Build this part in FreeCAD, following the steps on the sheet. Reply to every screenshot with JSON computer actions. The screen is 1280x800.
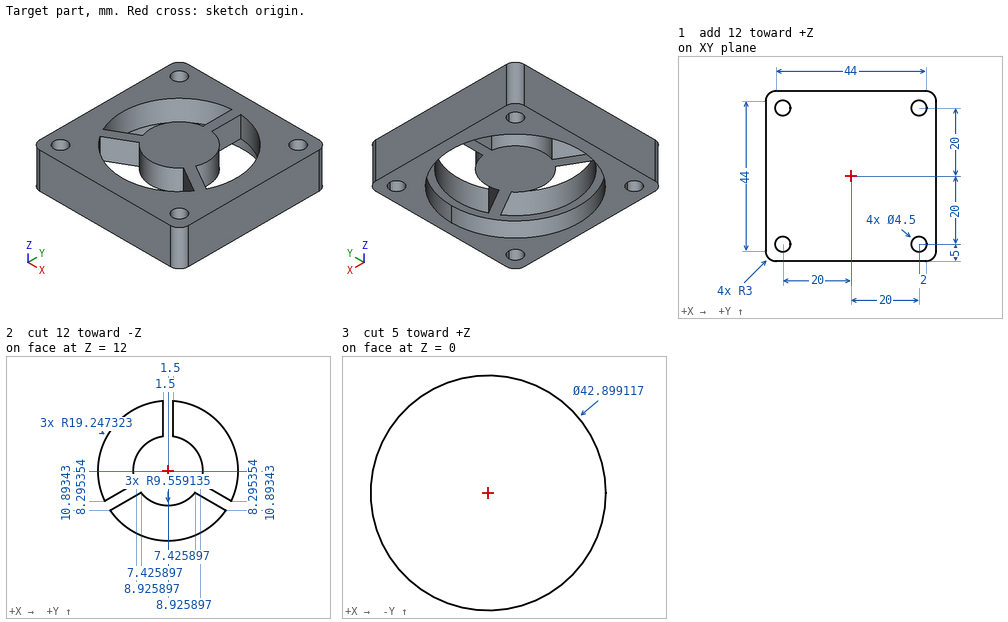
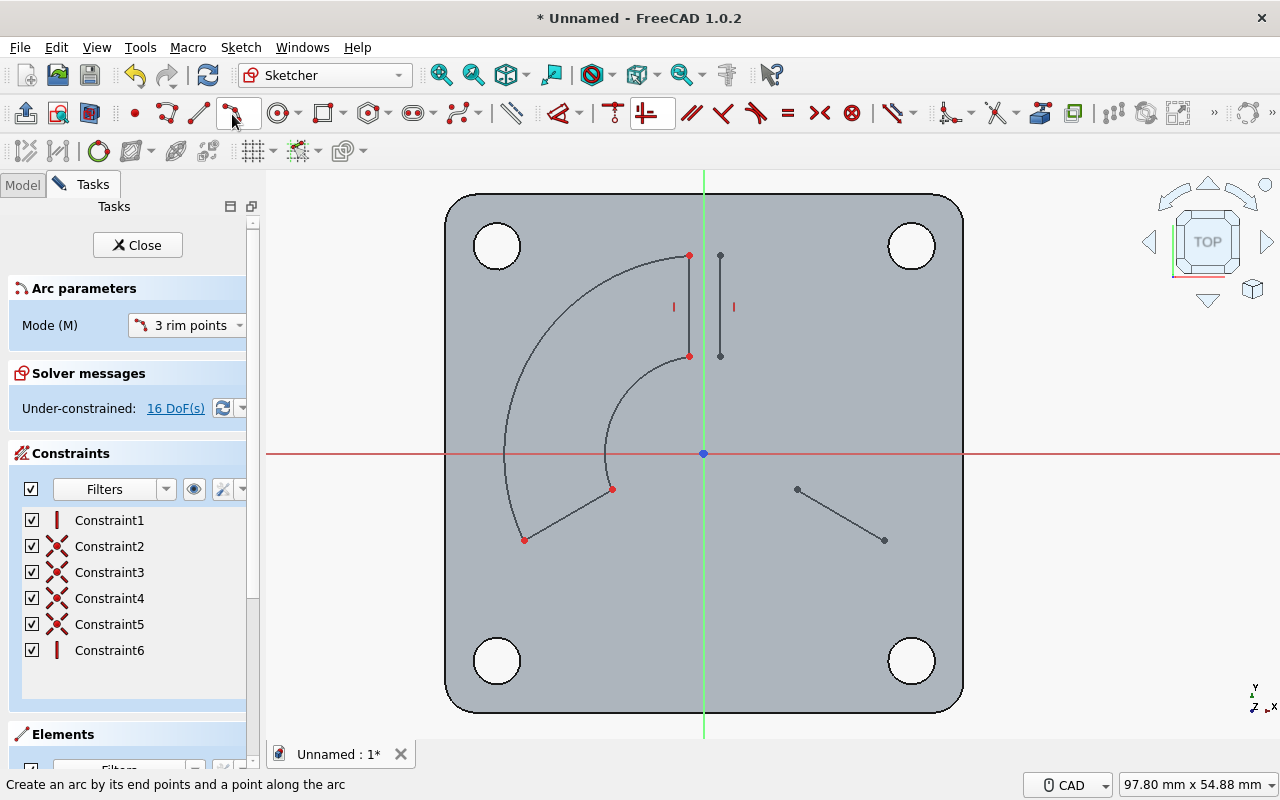
{"action": "left_click", "coordinate": [720, 357]}
{"action": "left_click", "coordinate": [797, 490]}
{"action": "left_click", "coordinate": [790, 404]}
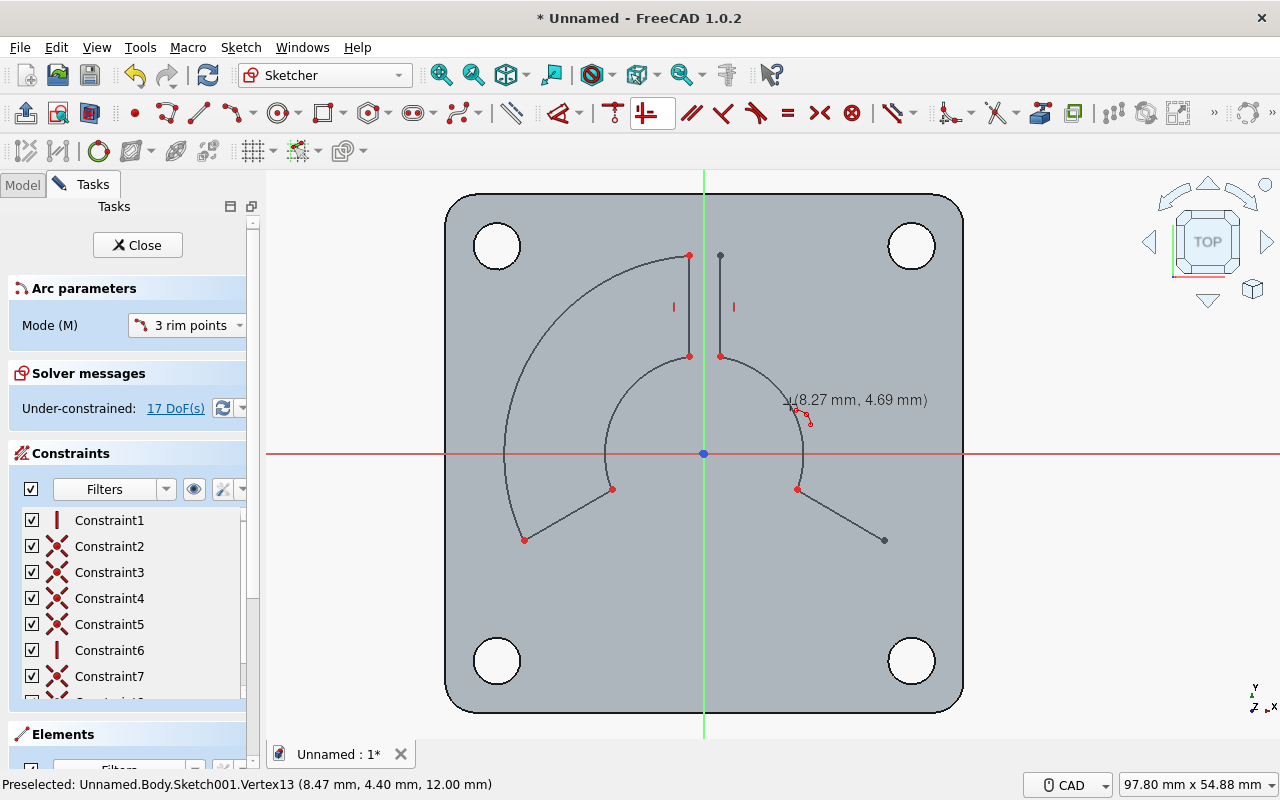
{"action": "left_click", "coordinate": [884, 541]}
{"action": "left_click", "coordinate": [720, 256]}
{"action": "left_click", "coordinate": [877, 354]}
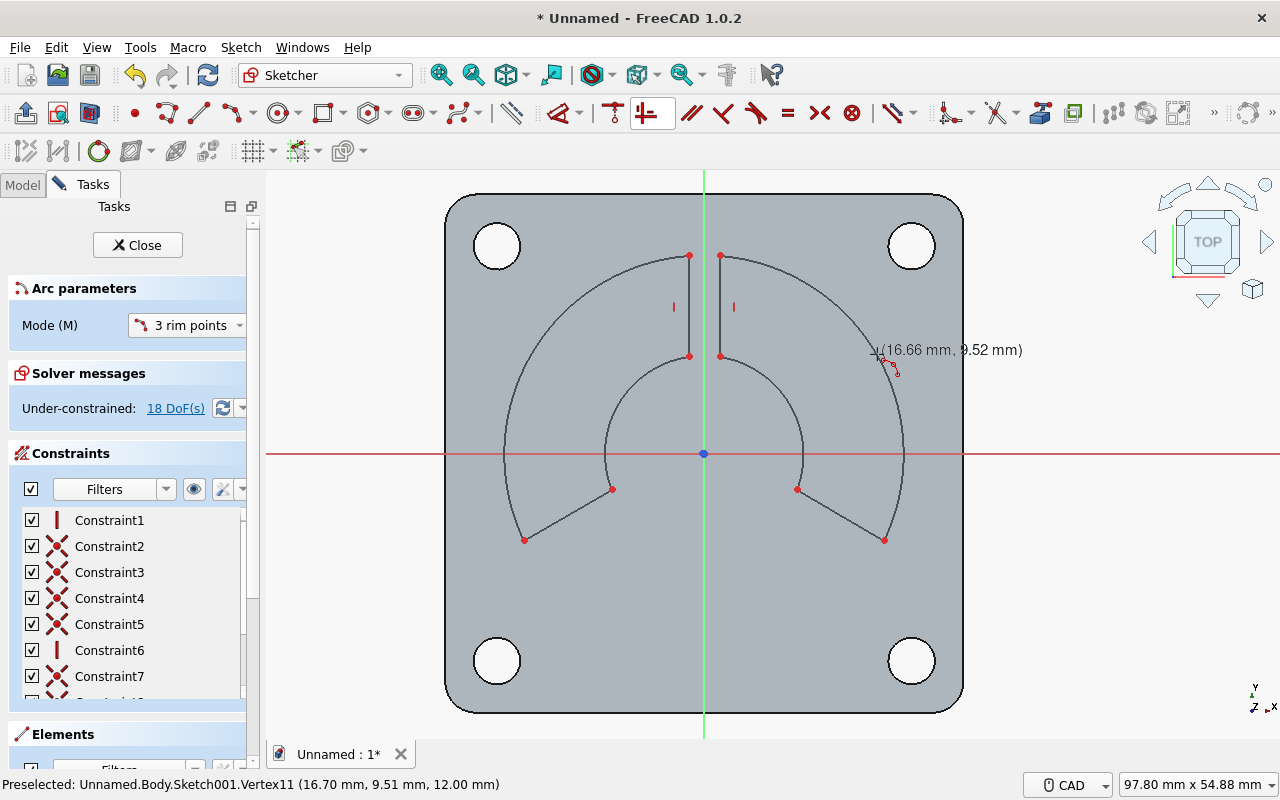
{"action": "left_click", "coordinate": [200, 114]}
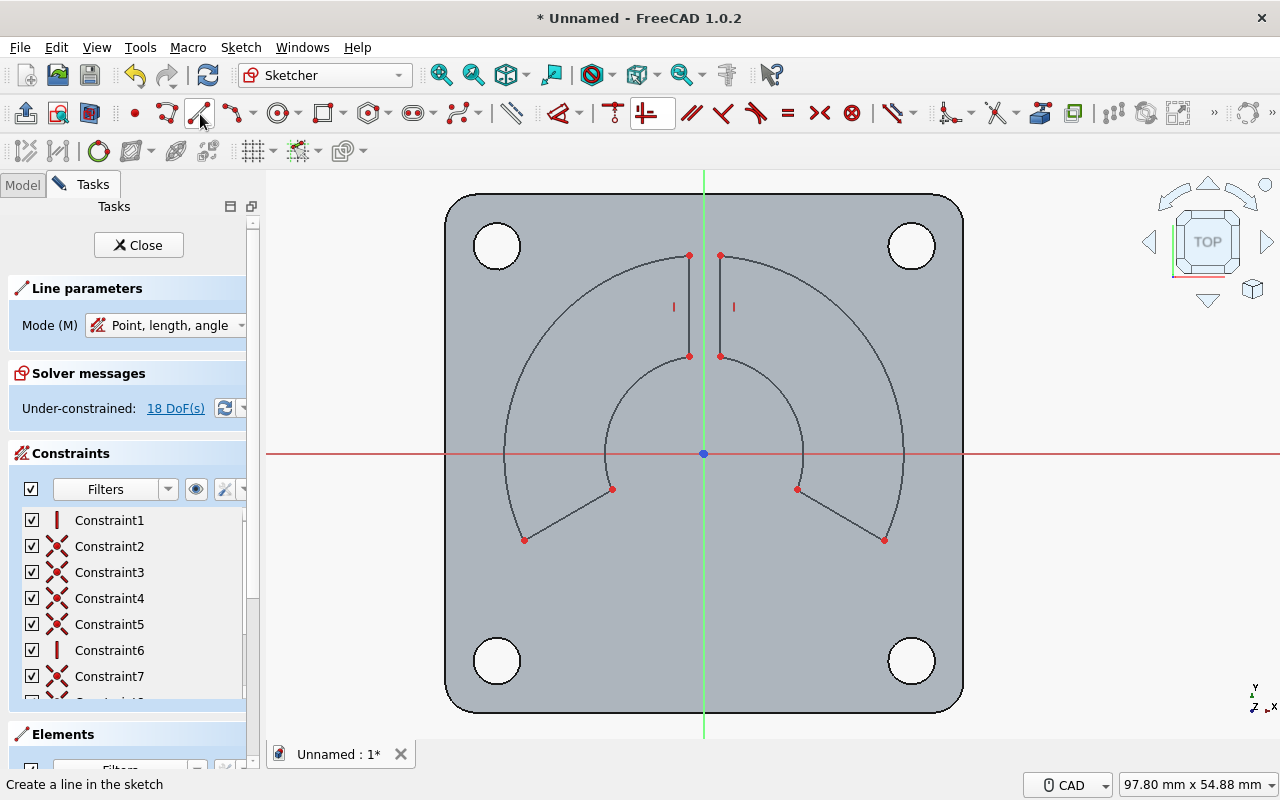
{"action": "left_click", "coordinate": [869, 567]}
{"action": "left_click", "coordinate": [781, 516]}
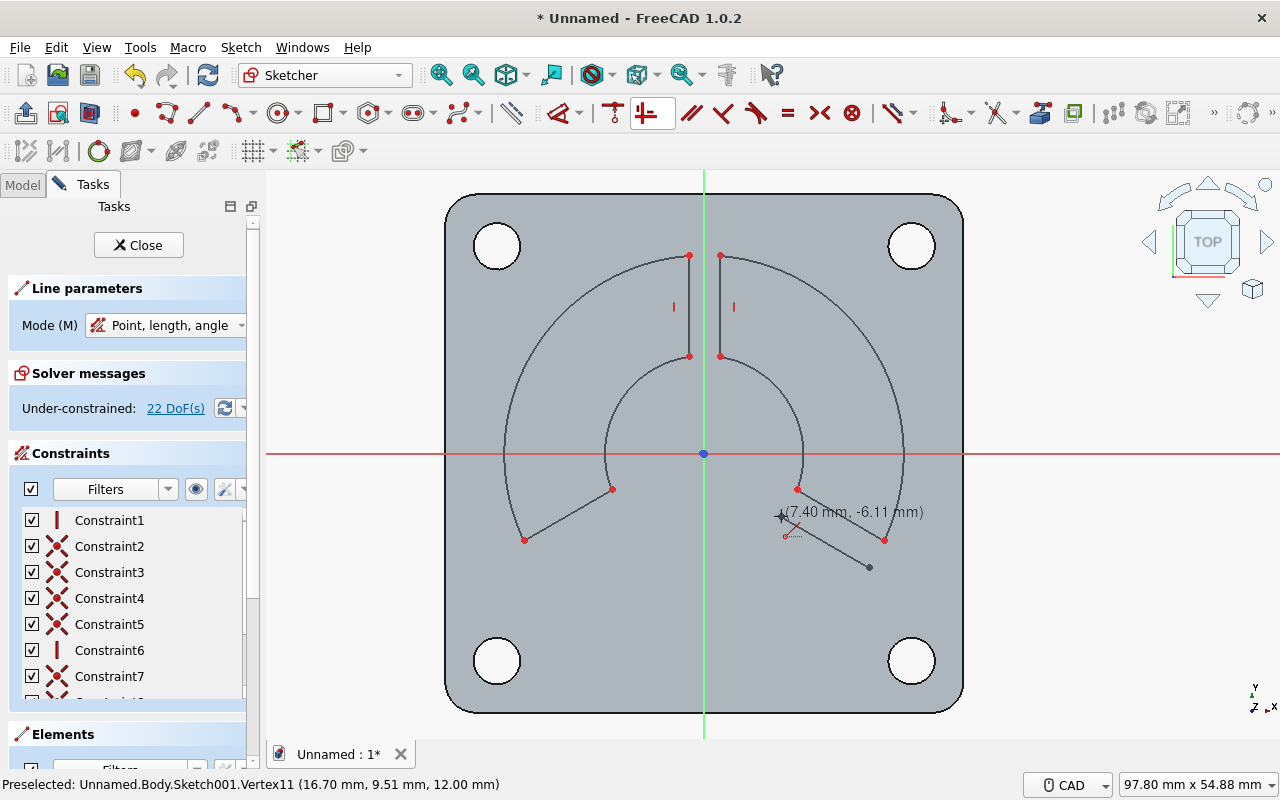
{"action": "left_click", "coordinate": [627, 516]}
{"action": "left_click", "coordinate": [540, 567]}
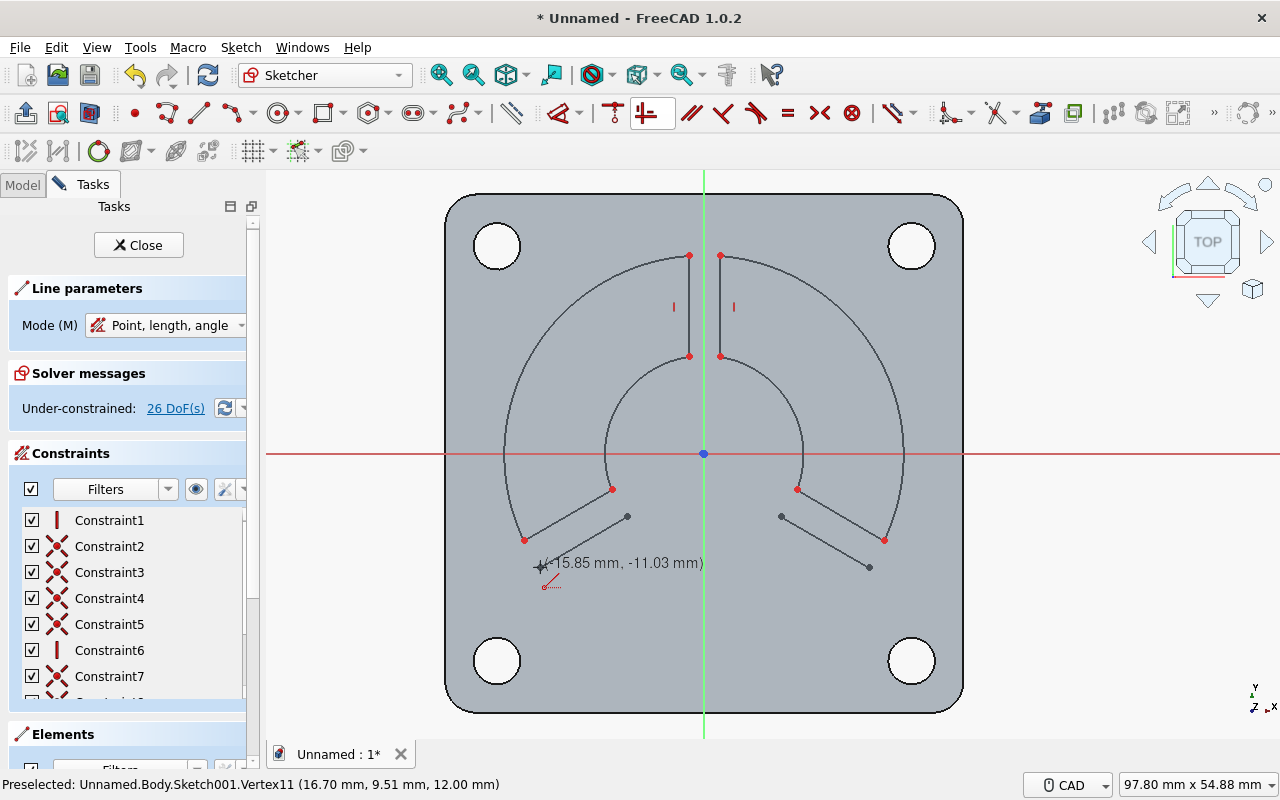
{"action": "left_click", "coordinate": [232, 114]}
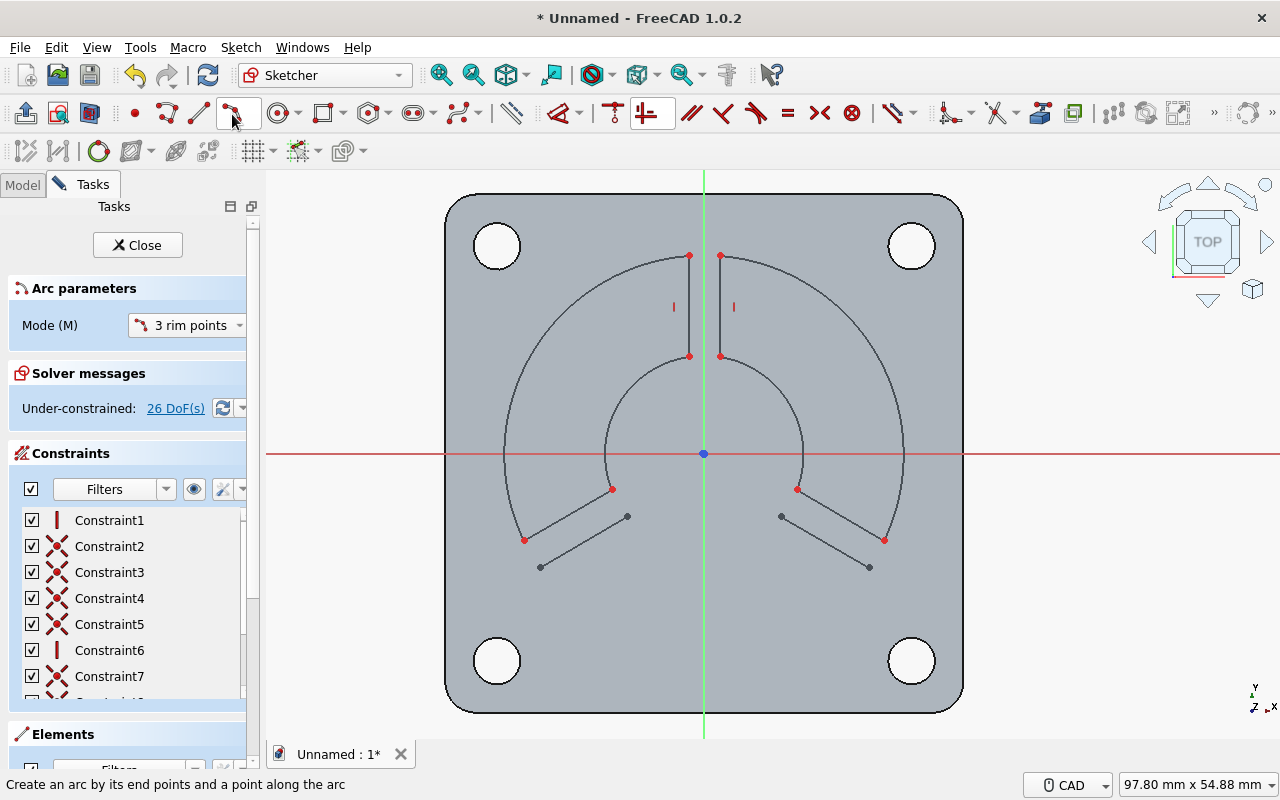
{"action": "left_click", "coordinate": [781, 517]}
{"action": "left_click", "coordinate": [627, 517]}
{"action": "left_click", "coordinate": [687, 551]}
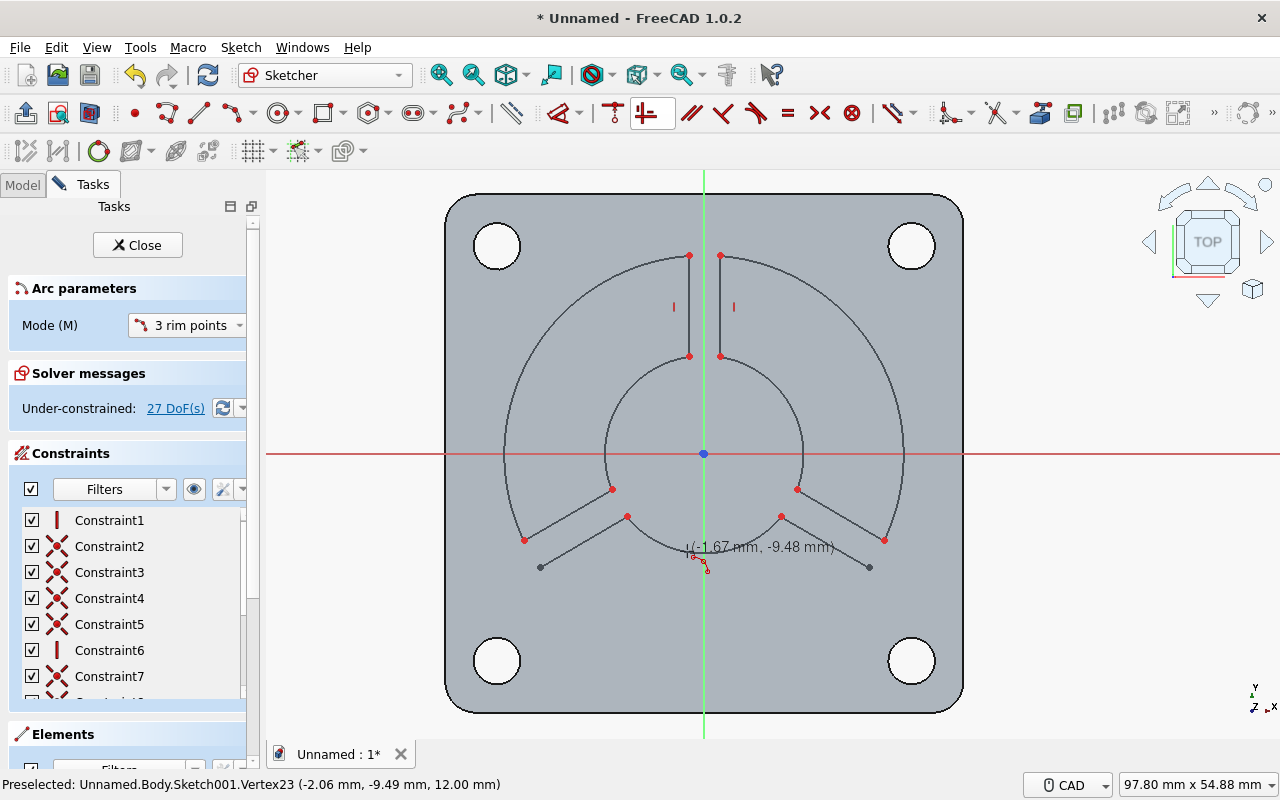
{"action": "left_click", "coordinate": [540, 568]}
{"action": "left_click", "coordinate": [869, 568]}
{"action": "left_click", "coordinate": [666, 649]}
{"action": "key", "text": "Escape"}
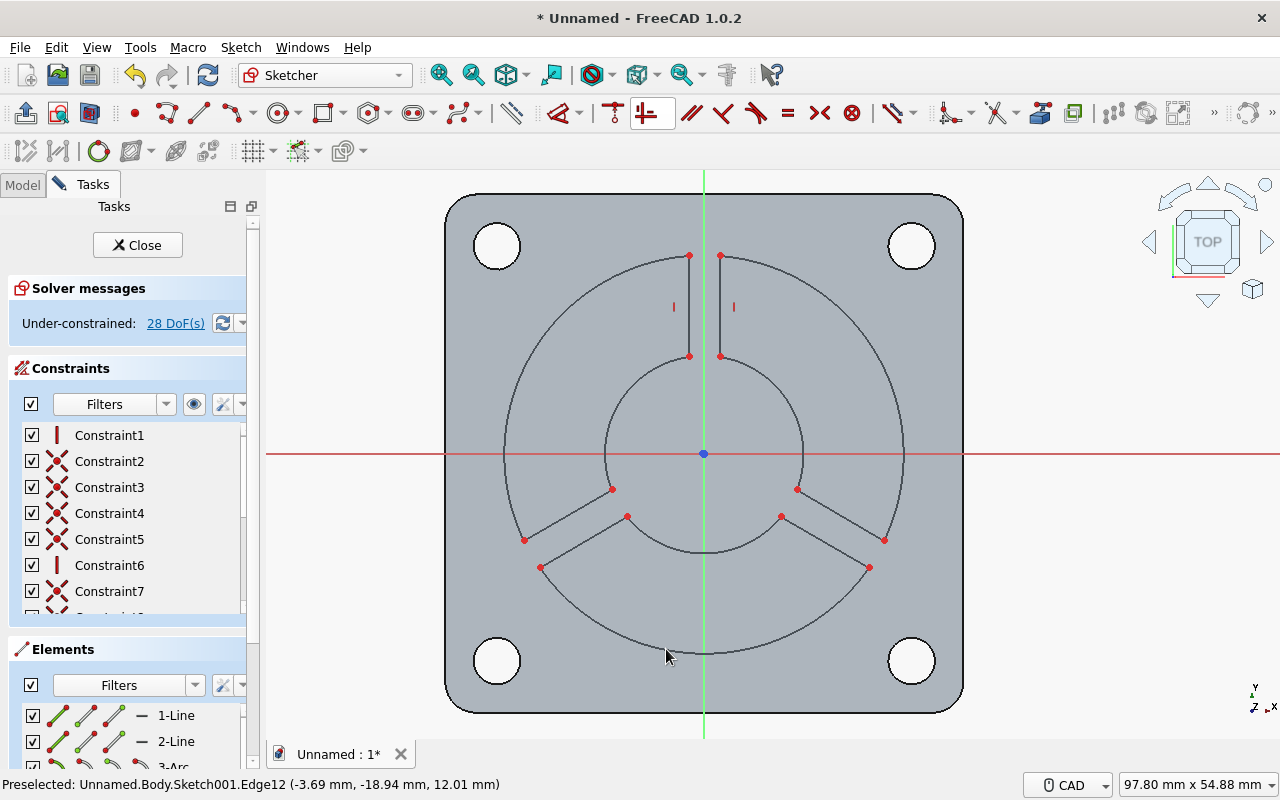
{"action": "left_click", "coordinate": [582, 297]}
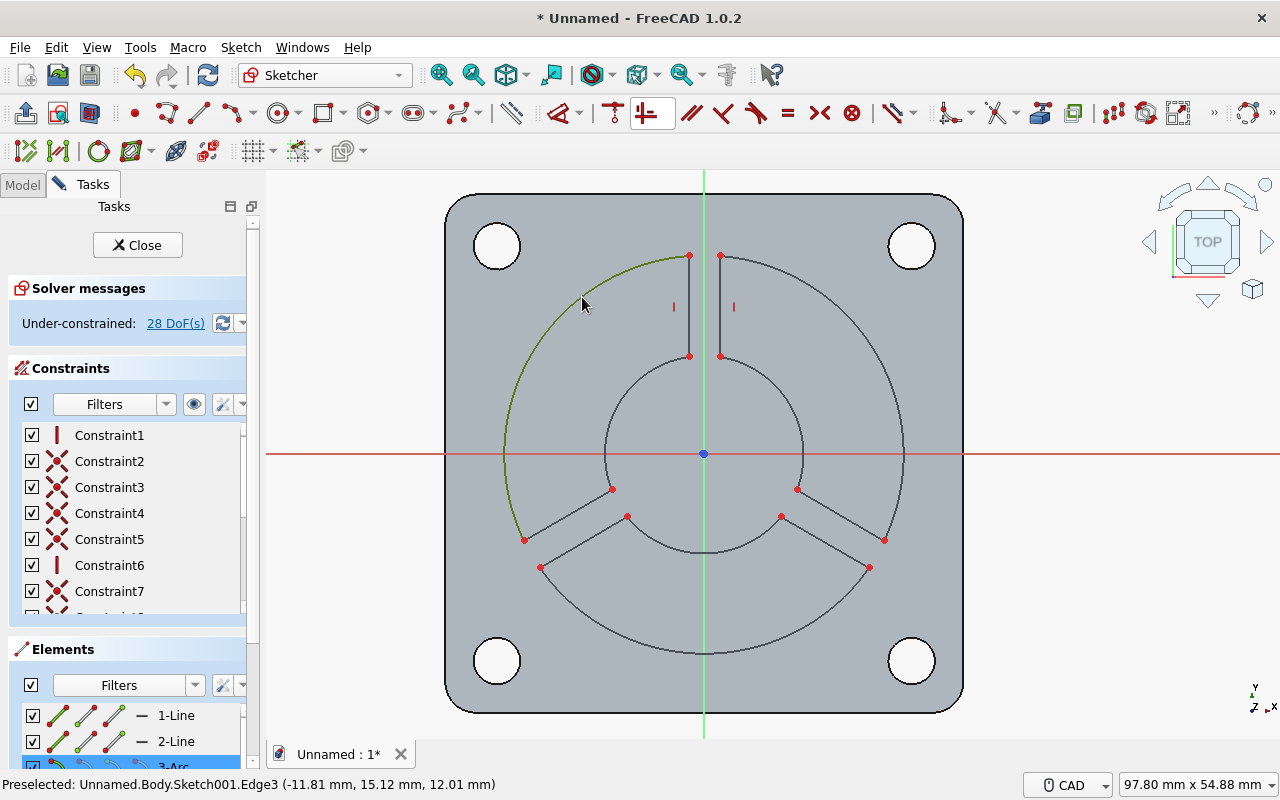
{"action": "left_click", "coordinate": [641, 378]}